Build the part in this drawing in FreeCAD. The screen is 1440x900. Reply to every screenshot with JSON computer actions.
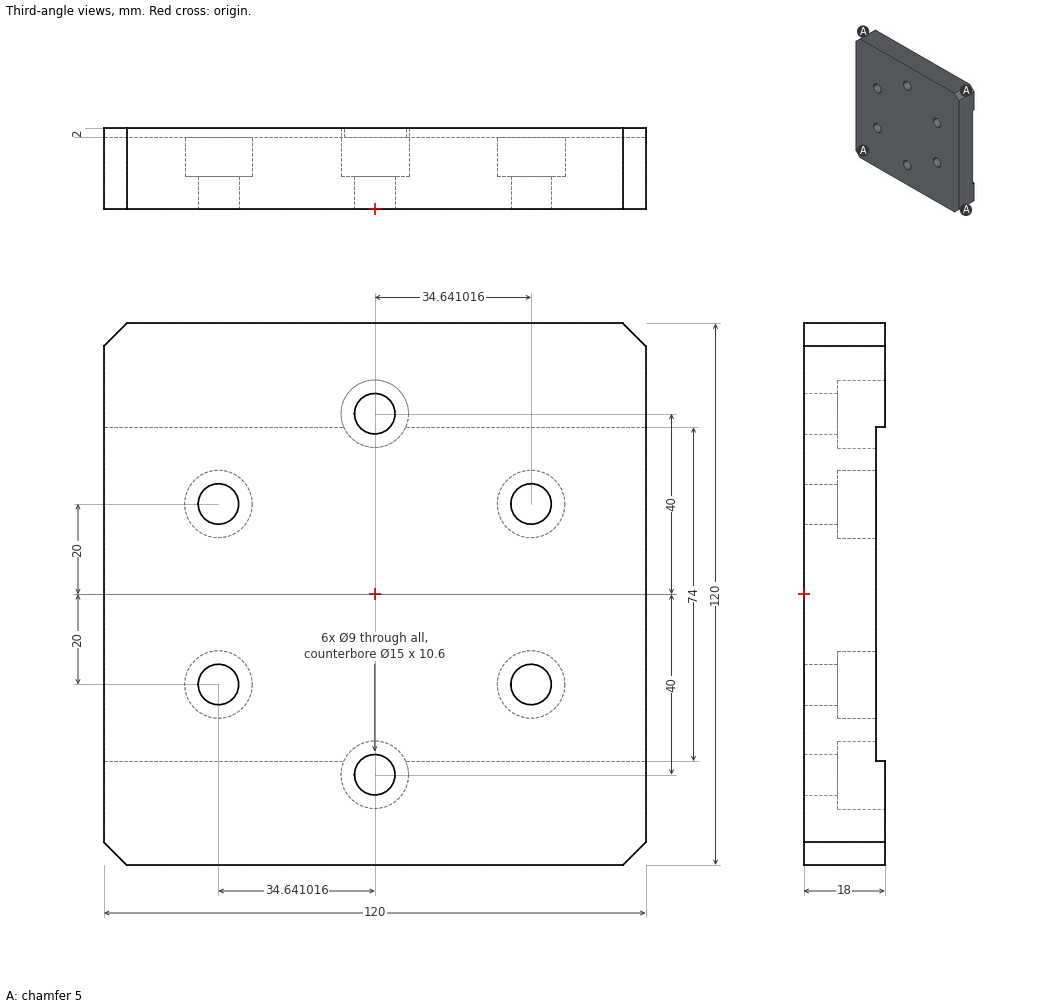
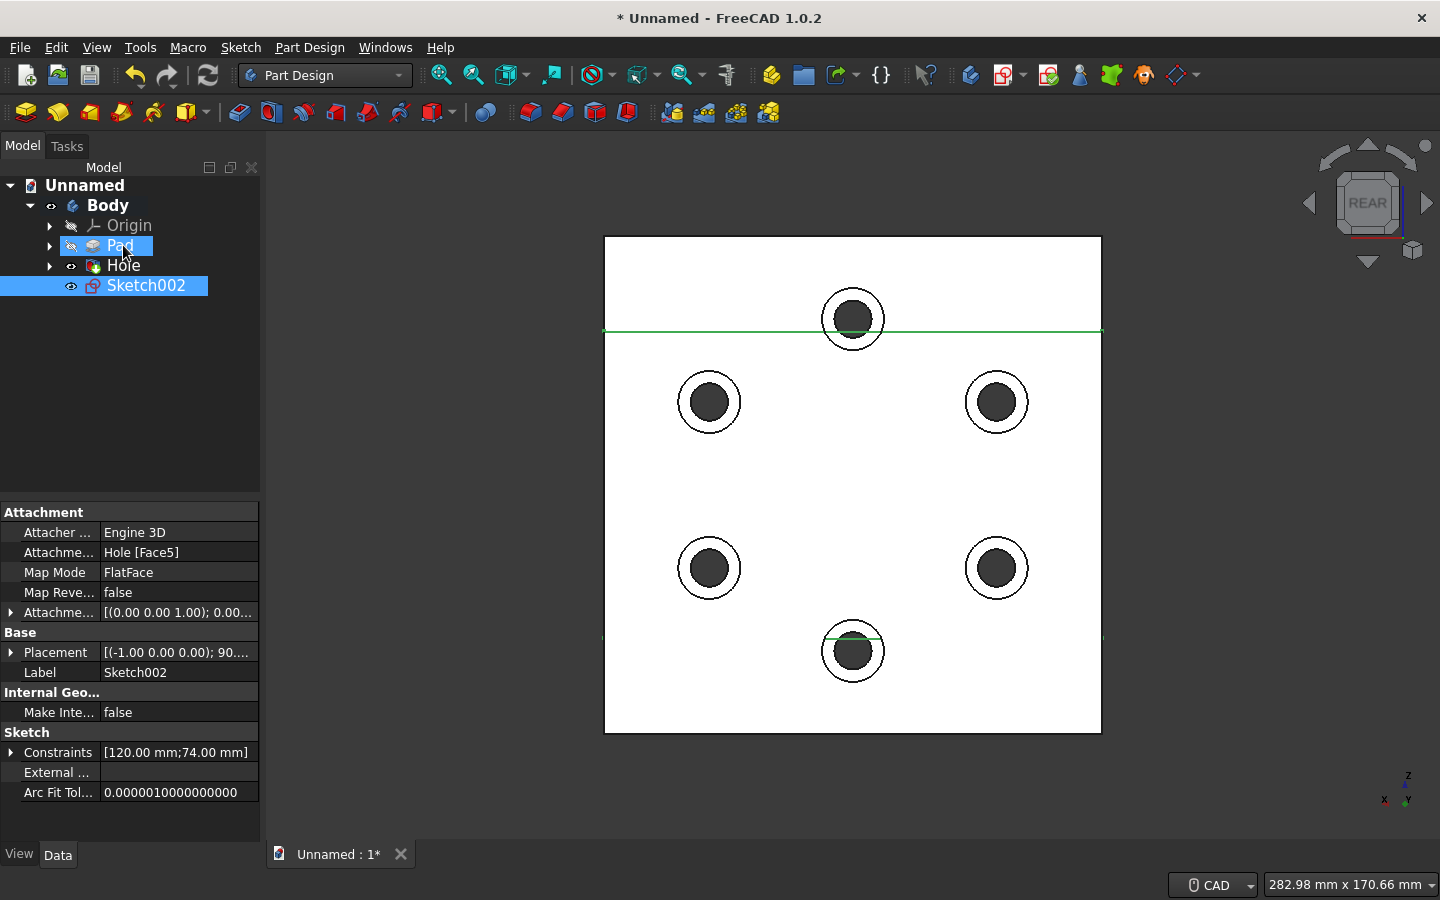
{"action": "left_click", "coordinate": [240, 112]}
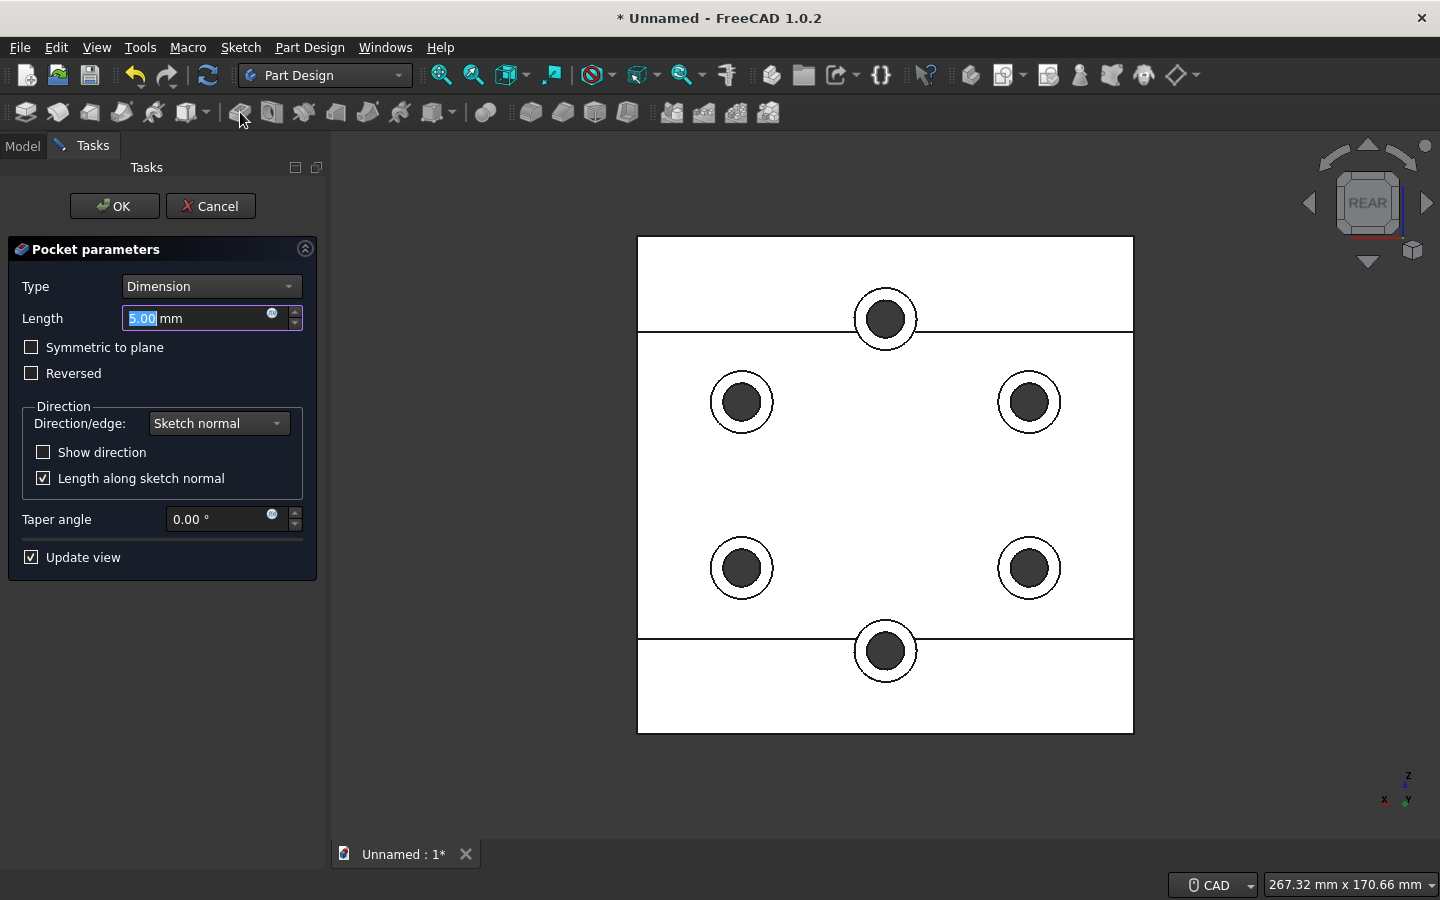
{"action": "type", "text": "2"}
{"action": "key", "text": "Tab"}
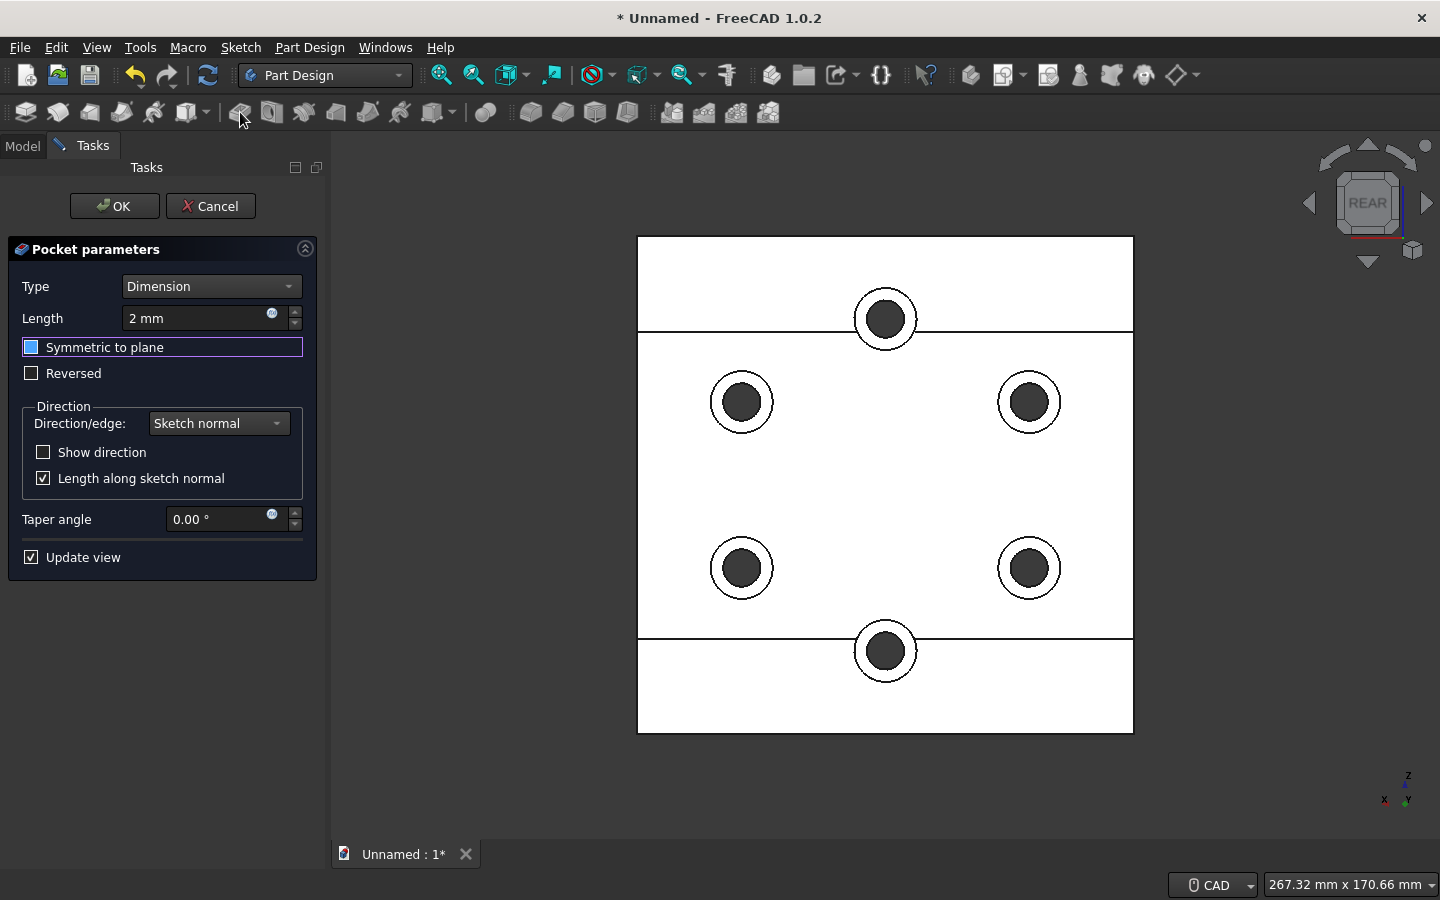
{"action": "left_click", "coordinate": [115, 206]}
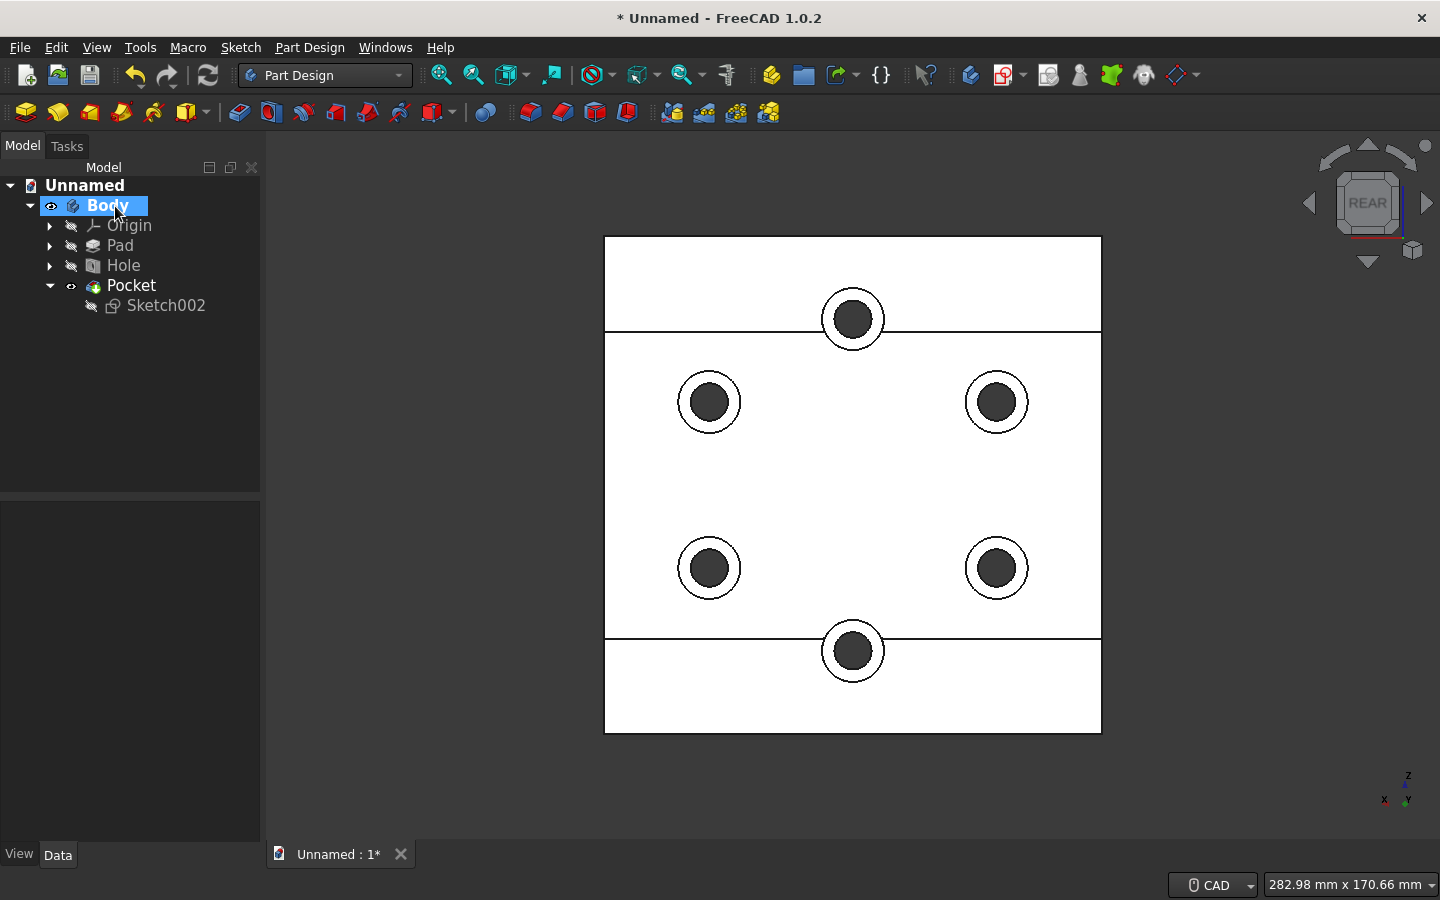
{"action": "key", "text": "0"}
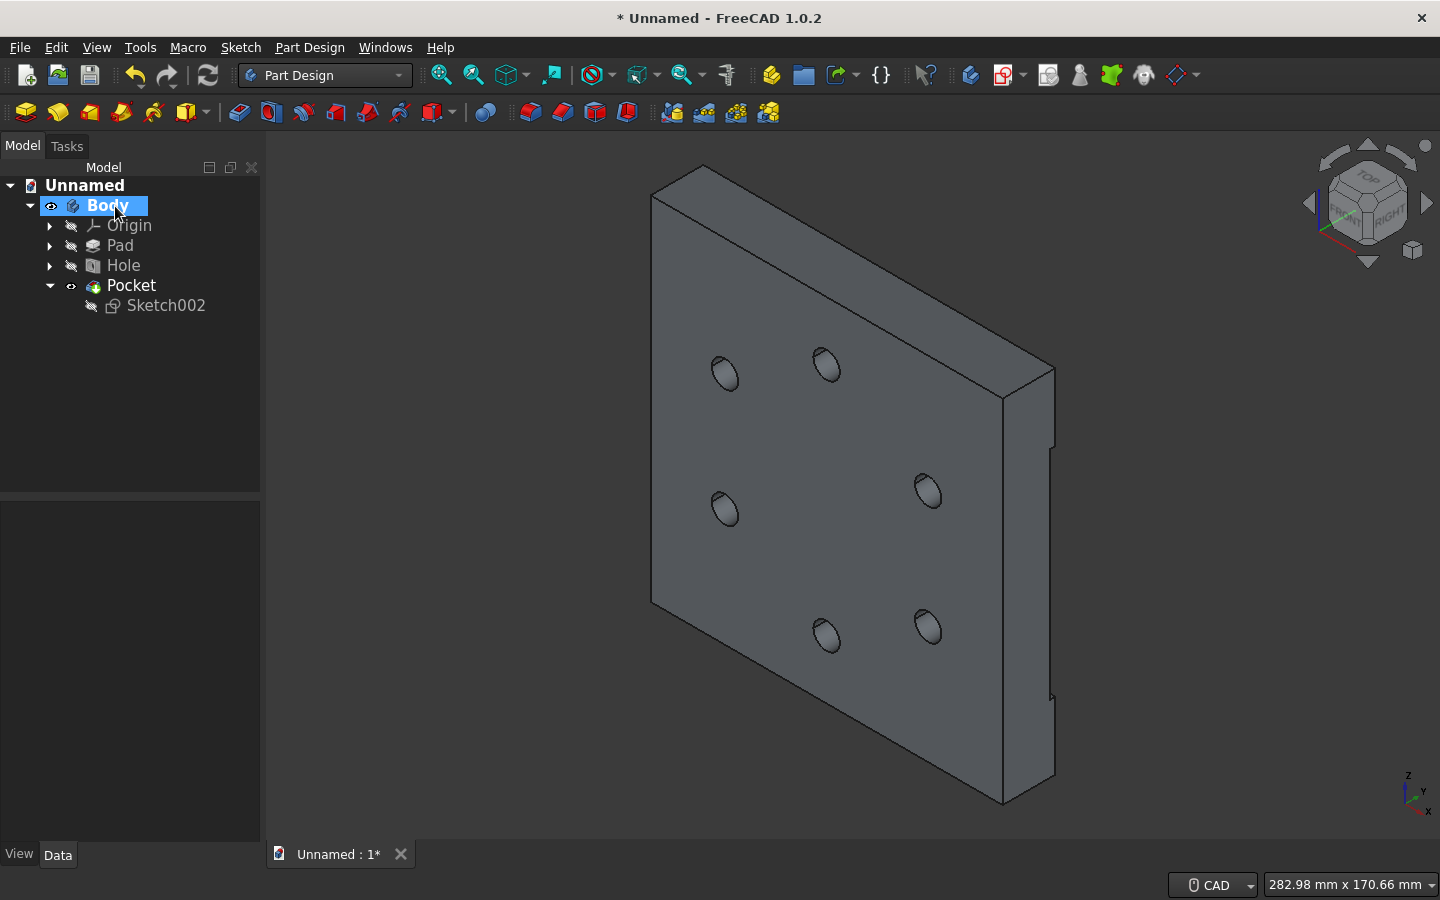
{"action": "left_click", "coordinate": [1029, 382]}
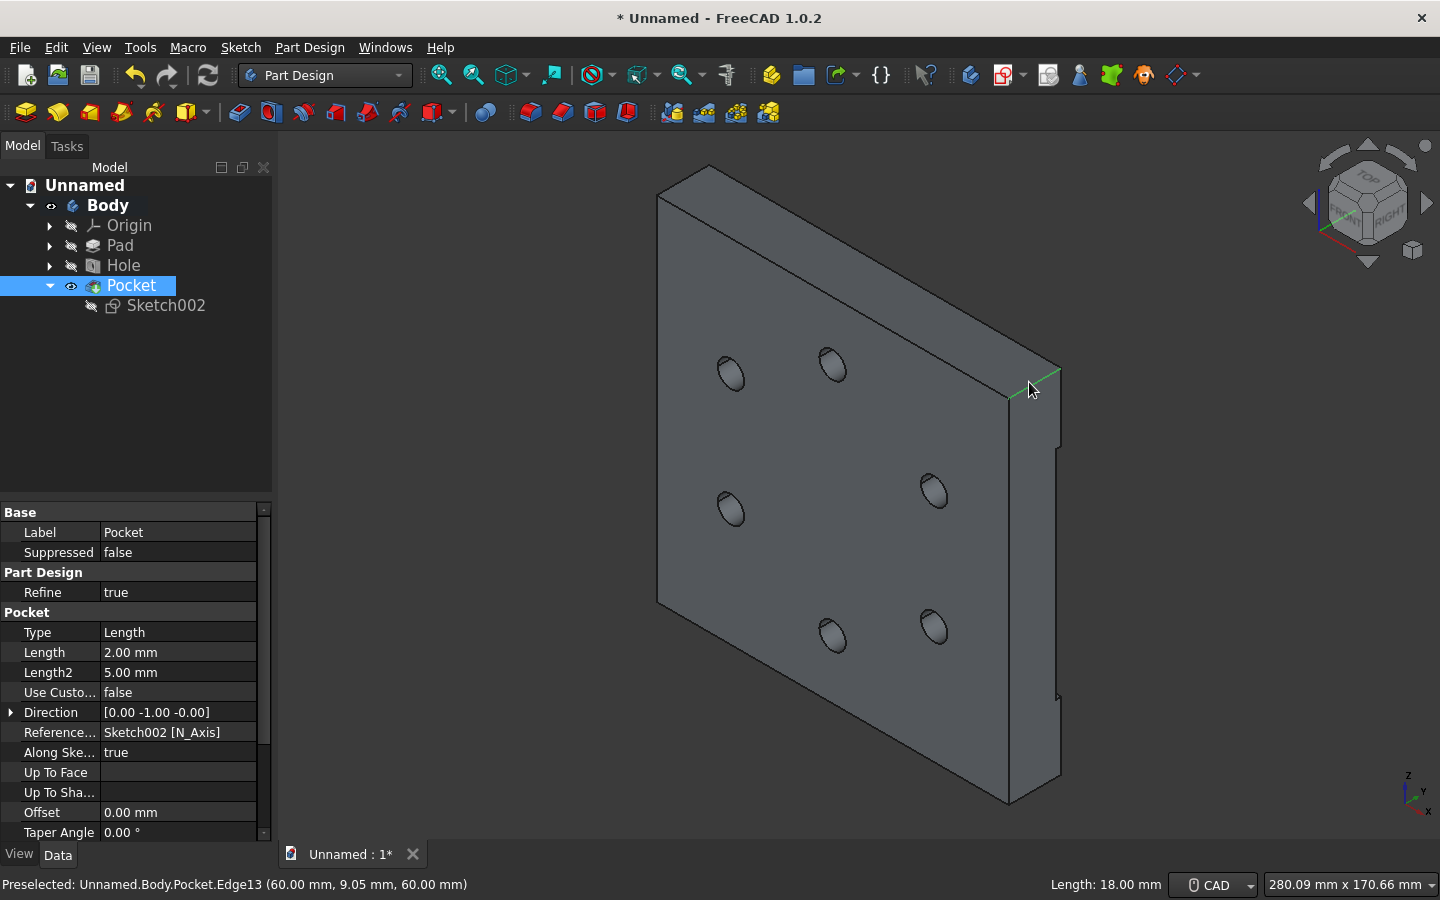
{"action": "key", "text": "2"}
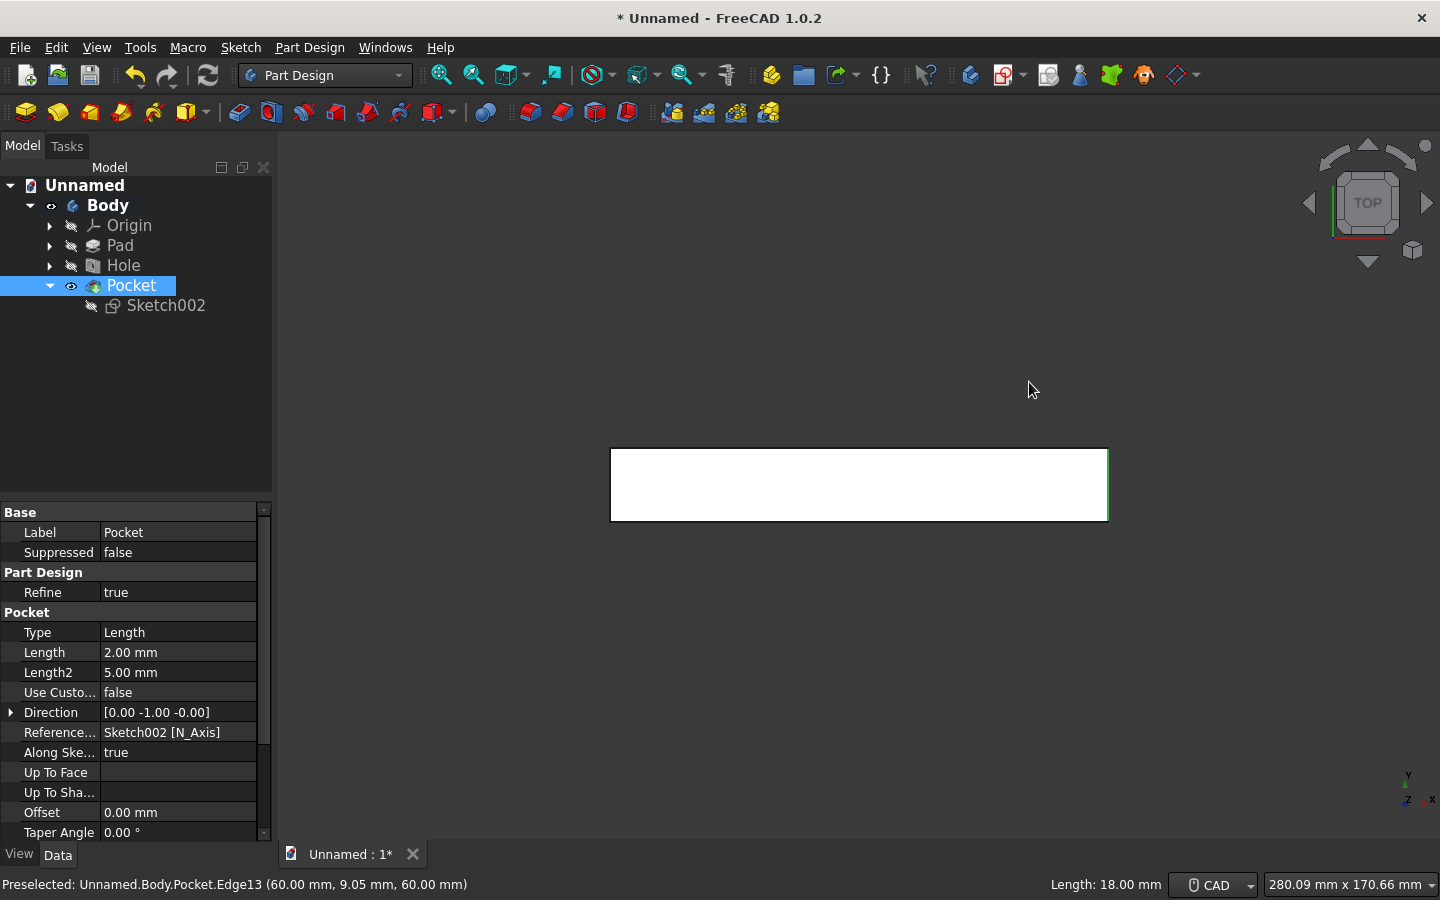
{"action": "left_click", "coordinate": [442, 76]}